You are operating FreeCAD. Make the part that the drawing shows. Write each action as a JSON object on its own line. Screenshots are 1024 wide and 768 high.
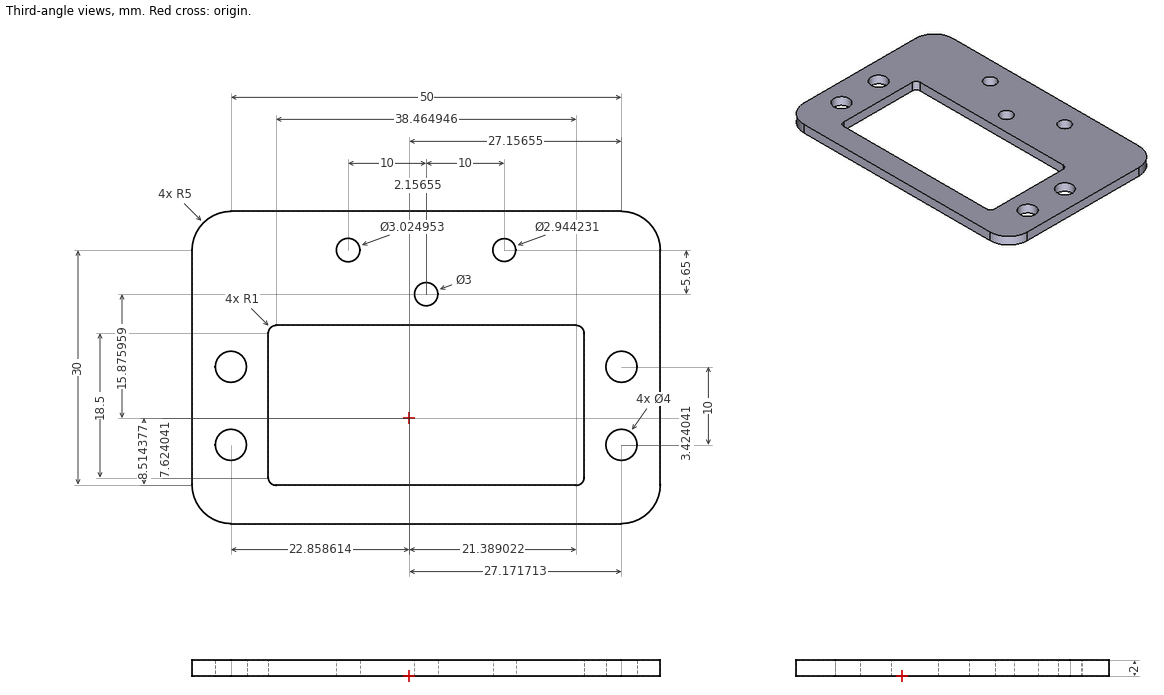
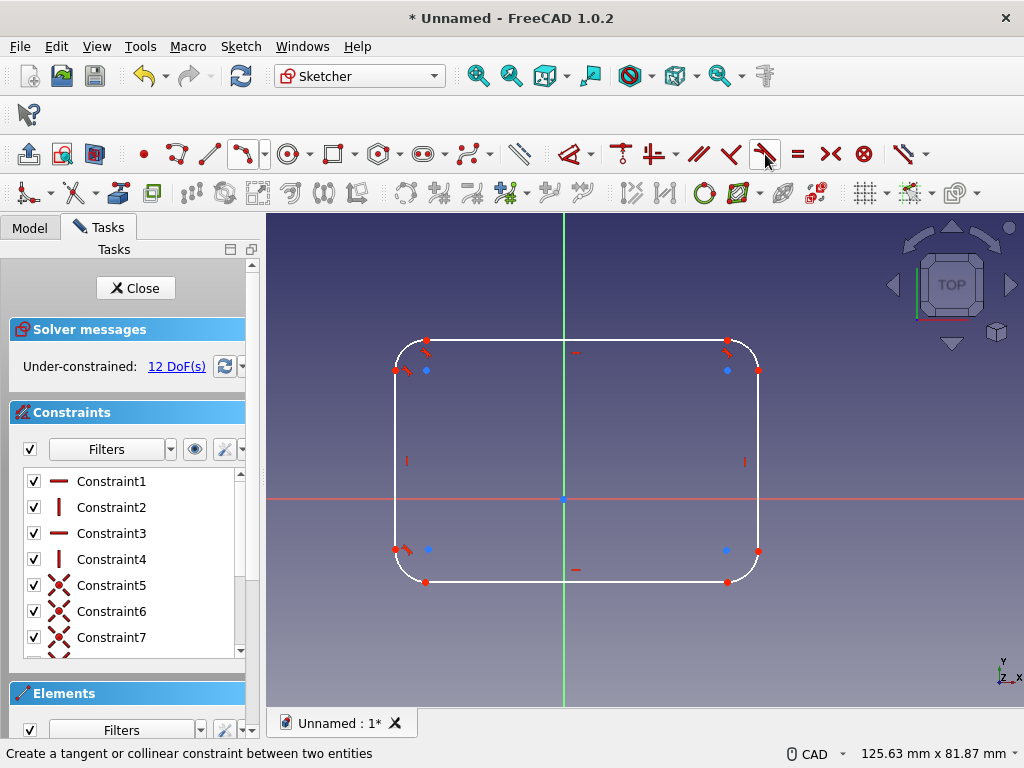
{"action": "left_click", "coordinate": [516, 582]}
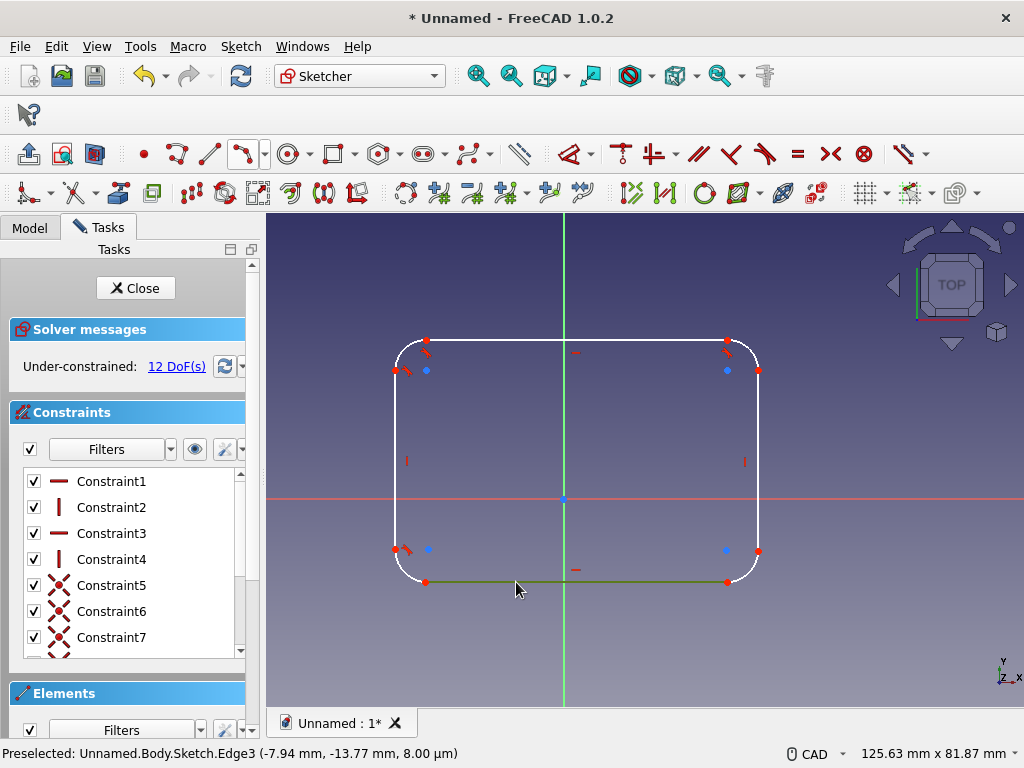
{"action": "left_click", "coordinate": [399, 564]}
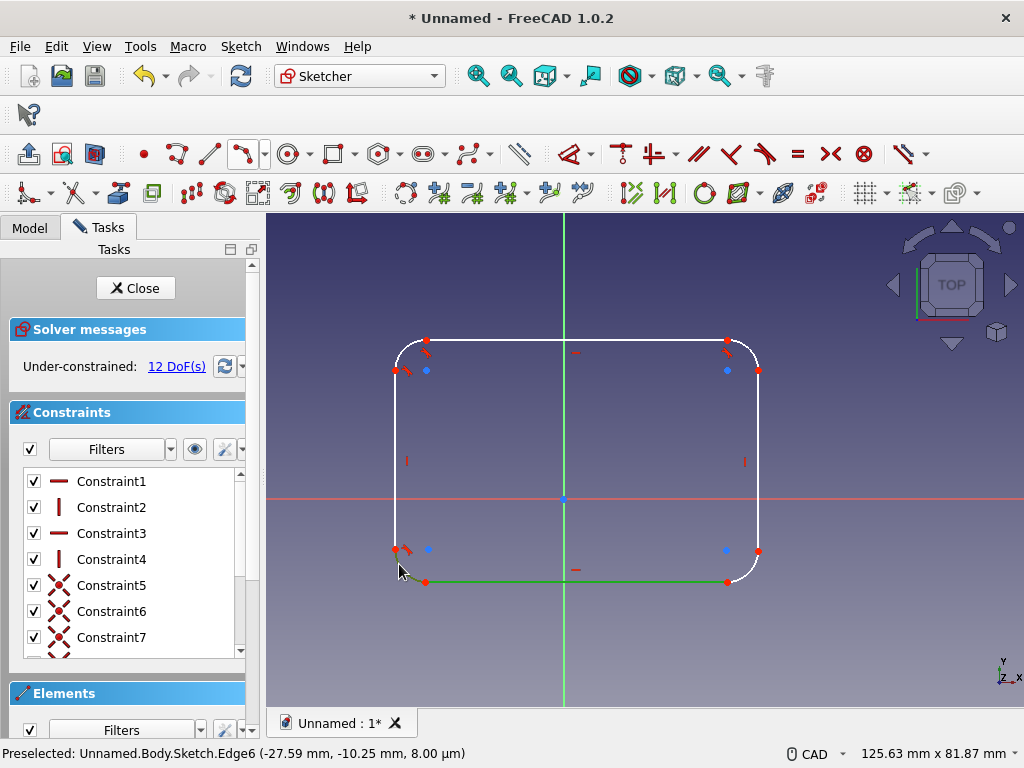
{"action": "left_click", "coordinate": [765, 154]}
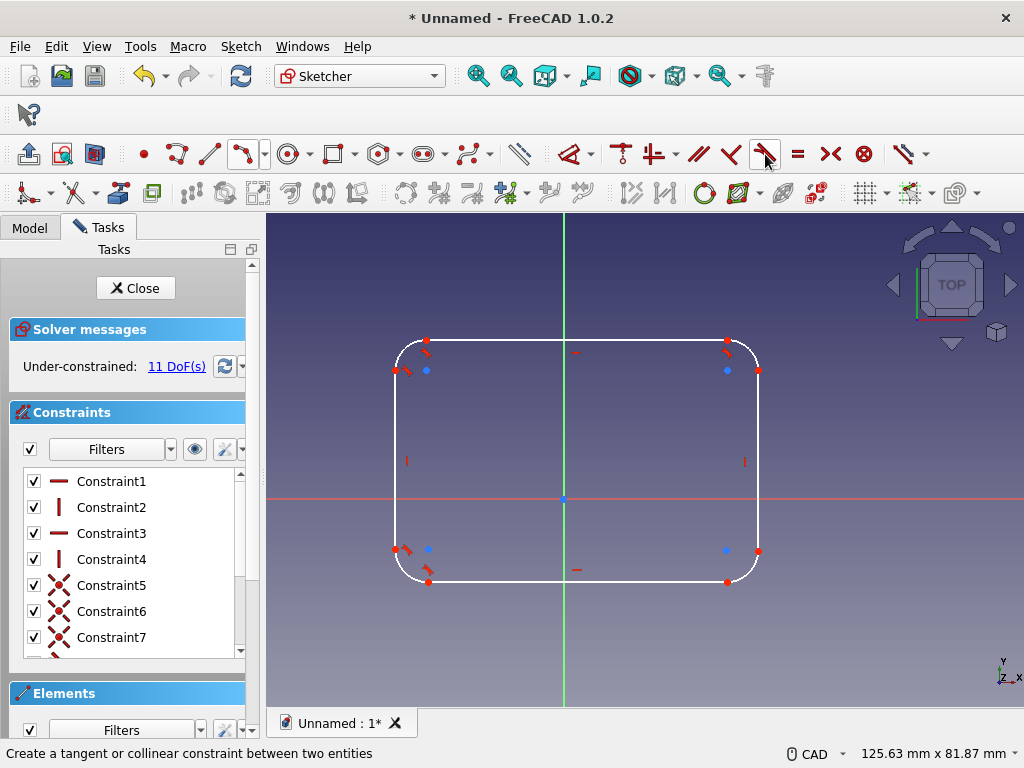
{"action": "left_click", "coordinate": [518, 582]}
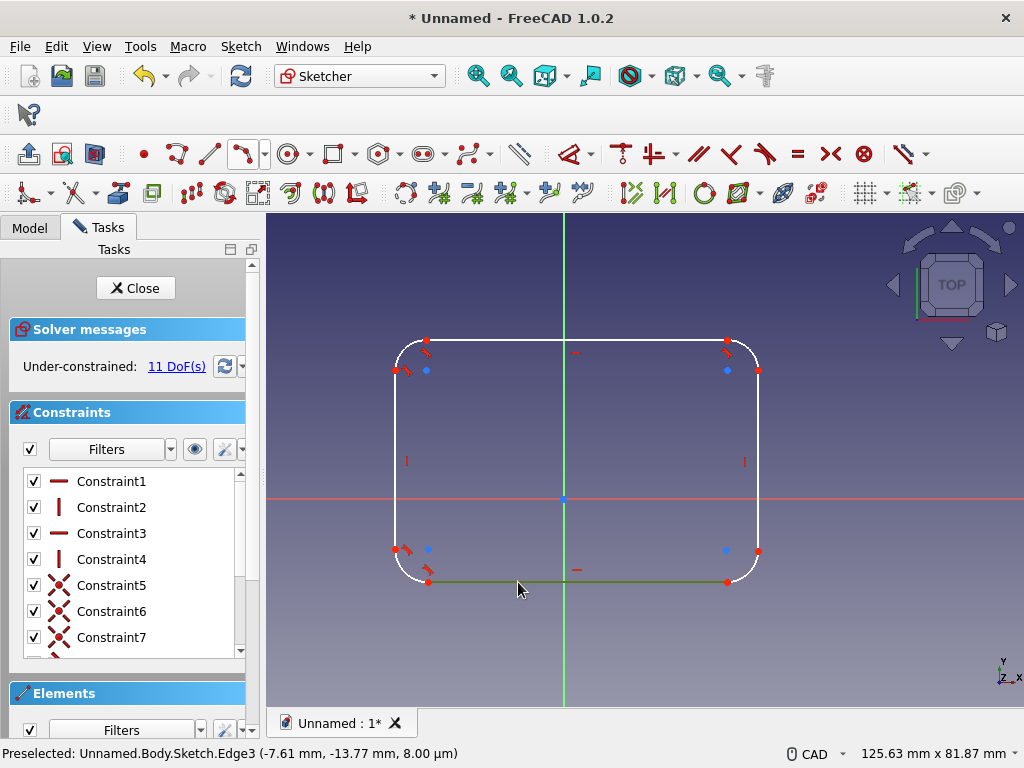
{"action": "left_click", "coordinate": [741, 578]}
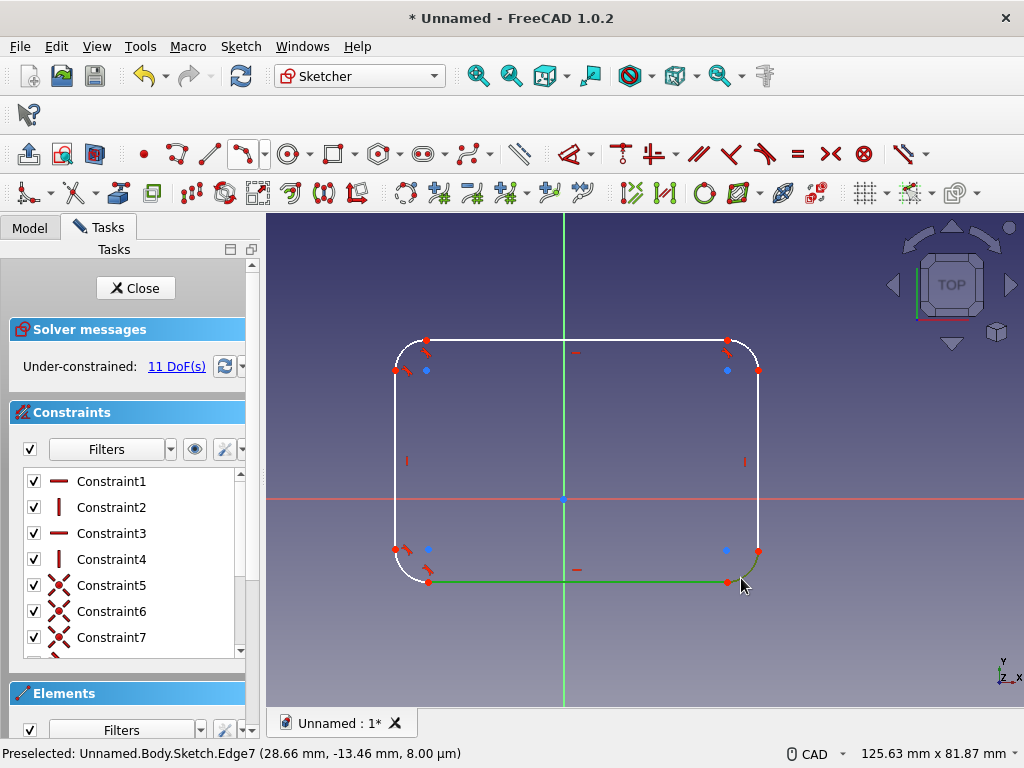
{"action": "key", "text": "t"}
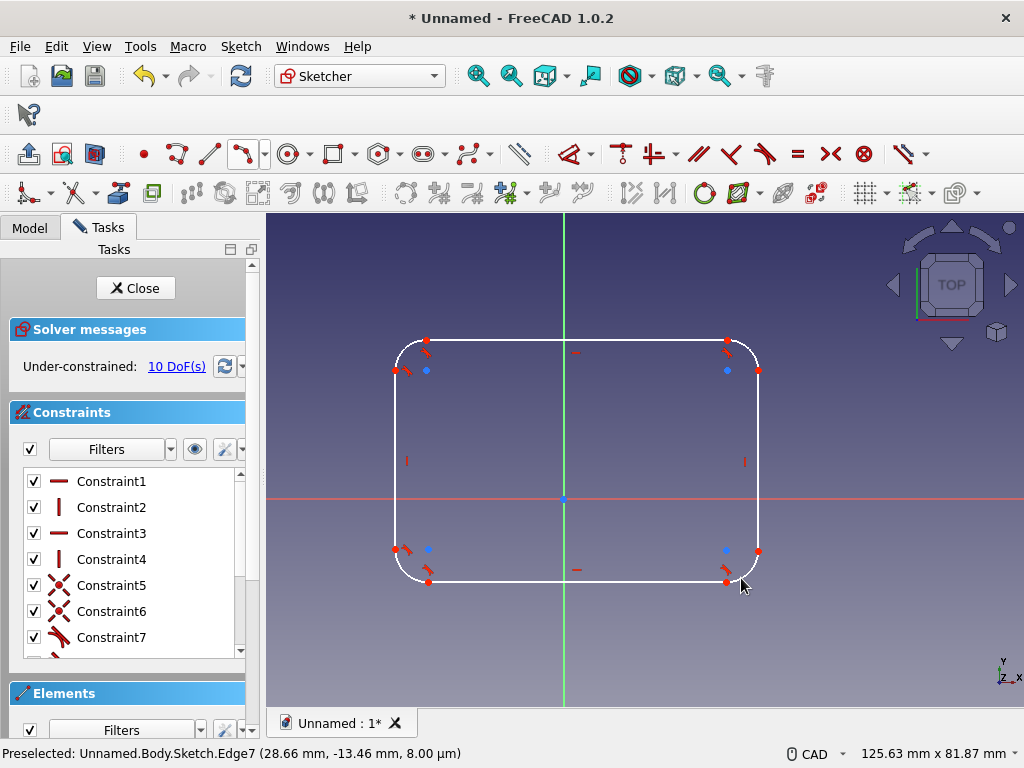
{"action": "left_click", "coordinate": [758, 497]}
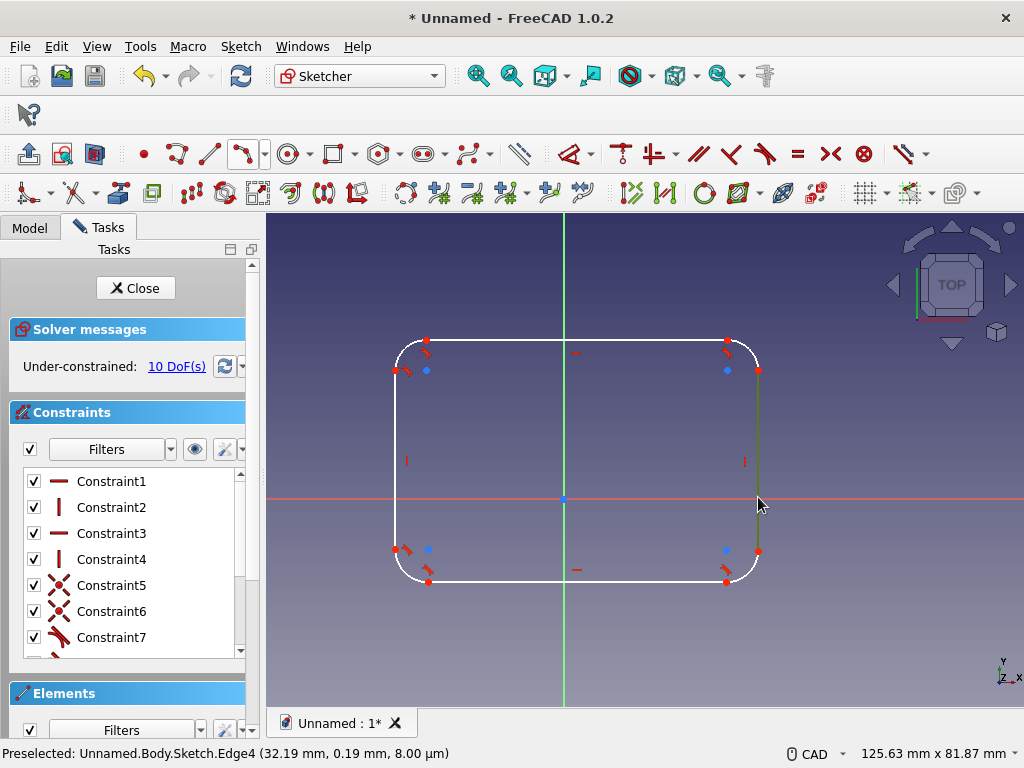
{"action": "left_click", "coordinate": [740, 579]}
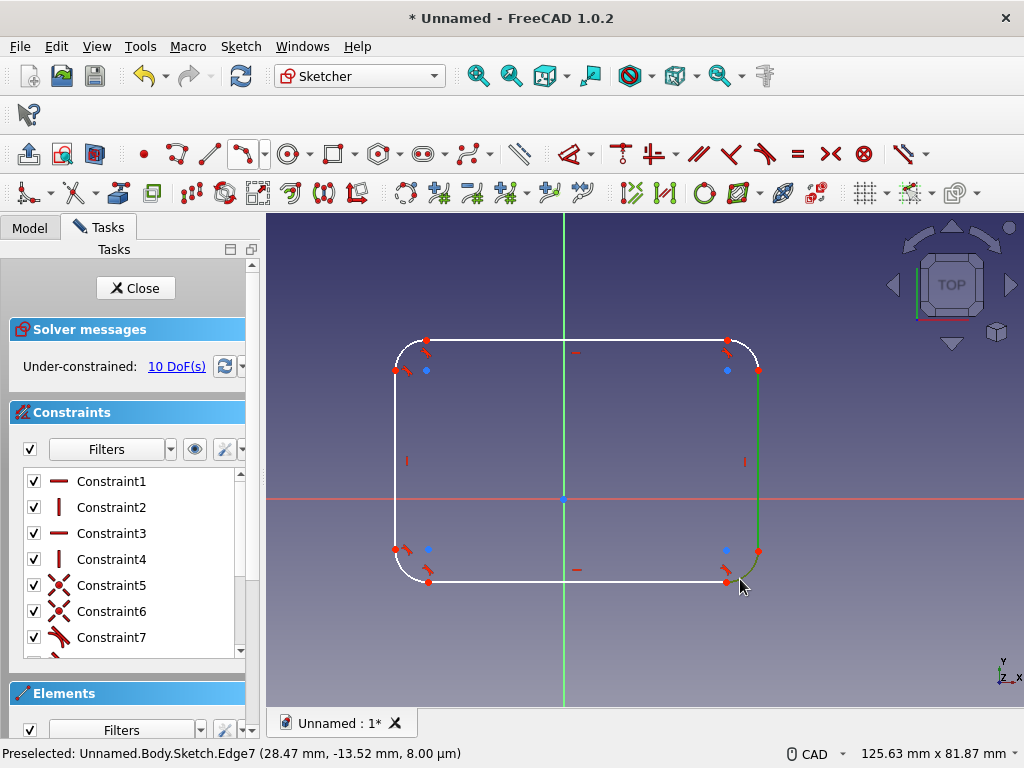
{"action": "key", "text": "t"}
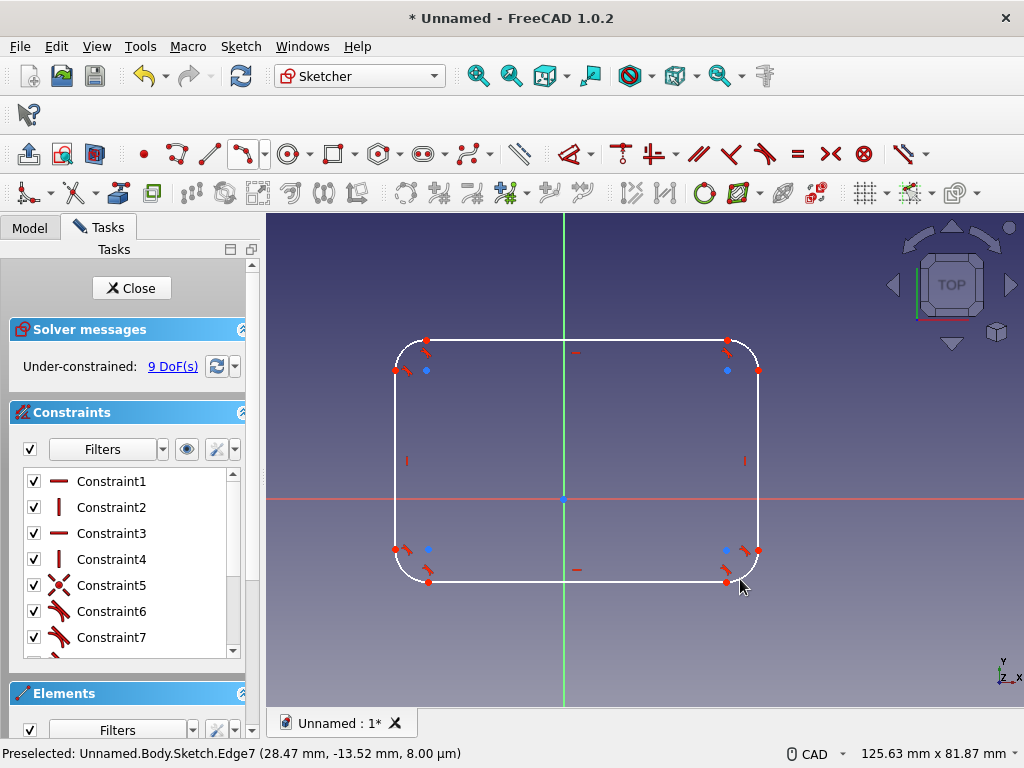
{"action": "left_click", "coordinate": [758, 496]}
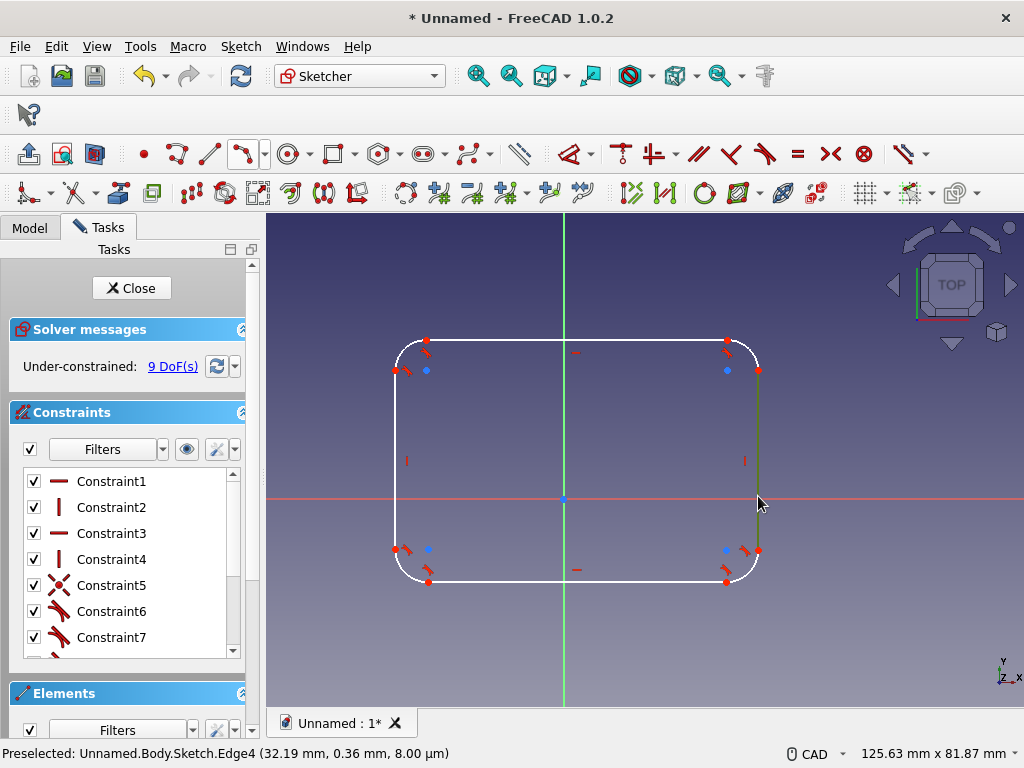
{"action": "left_click", "coordinate": [755, 357]}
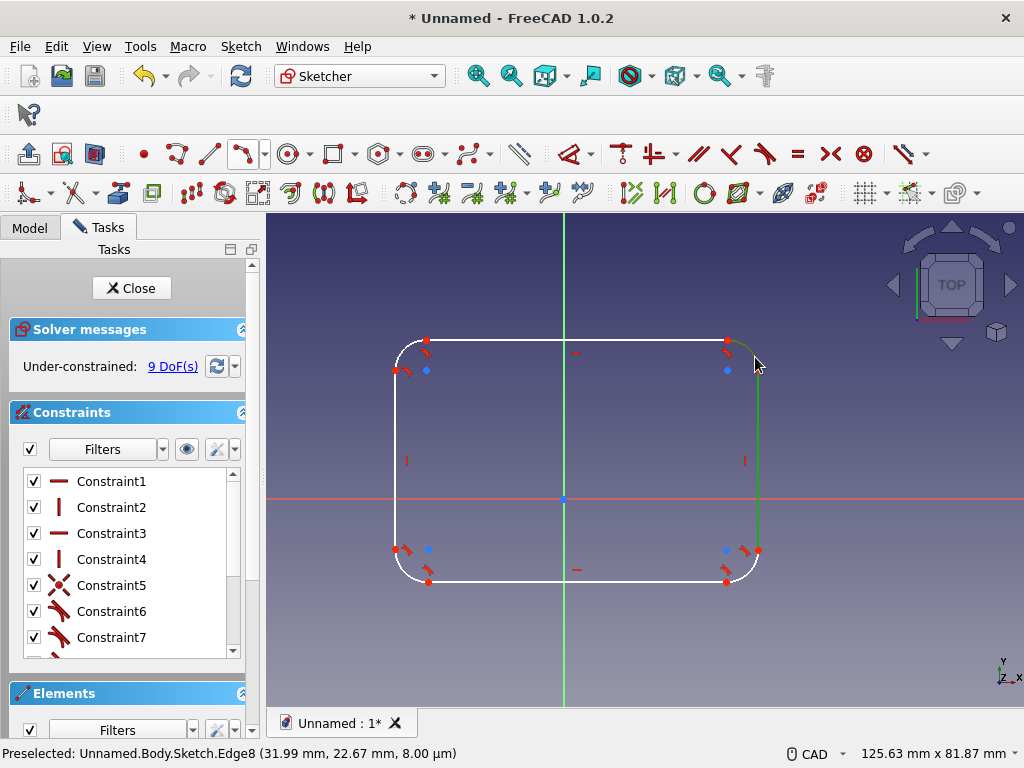
{"action": "left_click", "coordinate": [765, 154]}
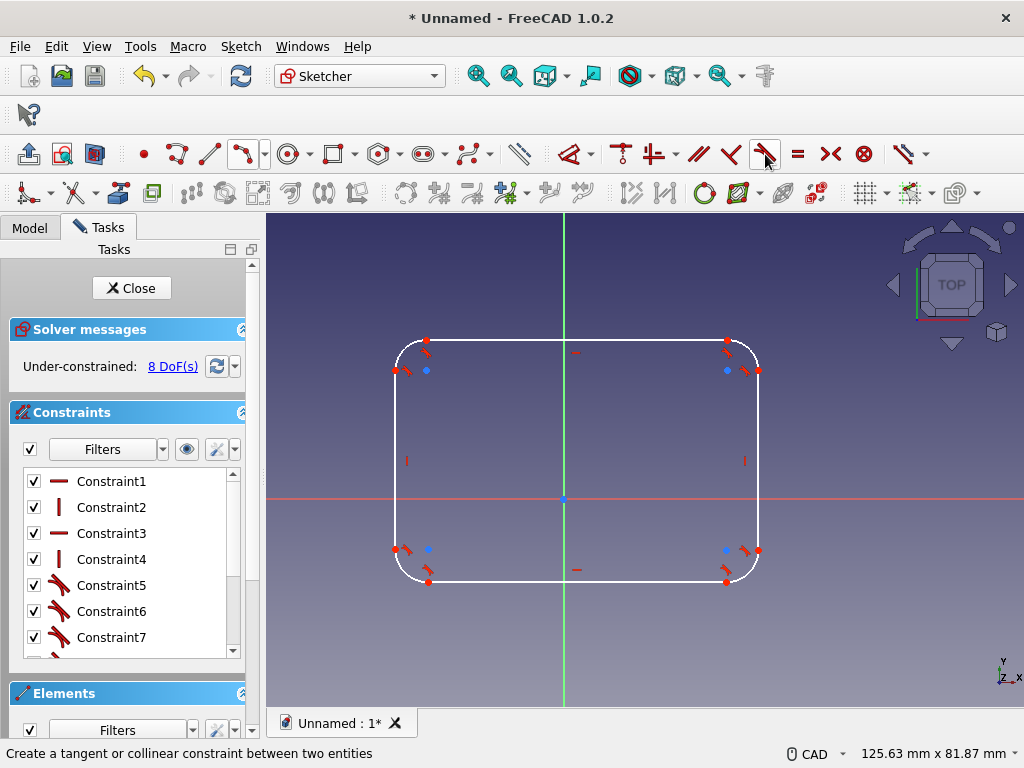
{"action": "left_click", "coordinate": [412, 344]}